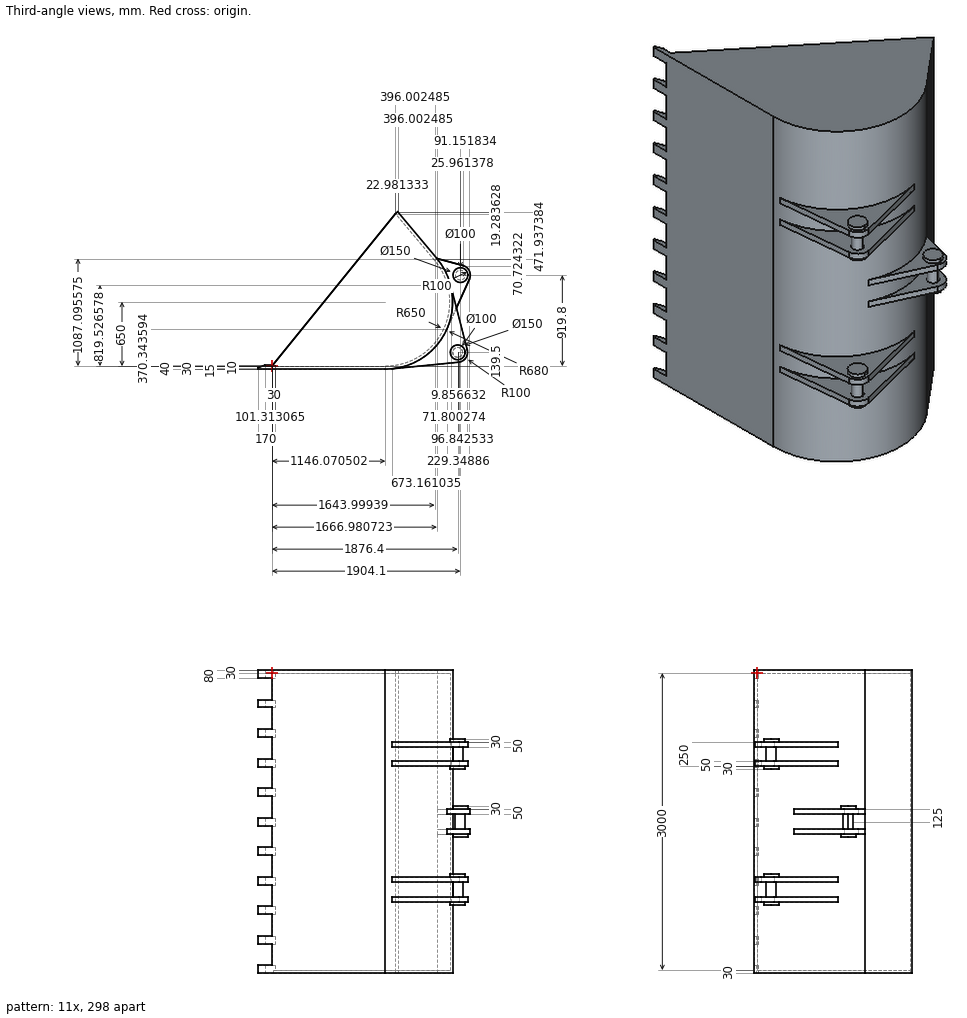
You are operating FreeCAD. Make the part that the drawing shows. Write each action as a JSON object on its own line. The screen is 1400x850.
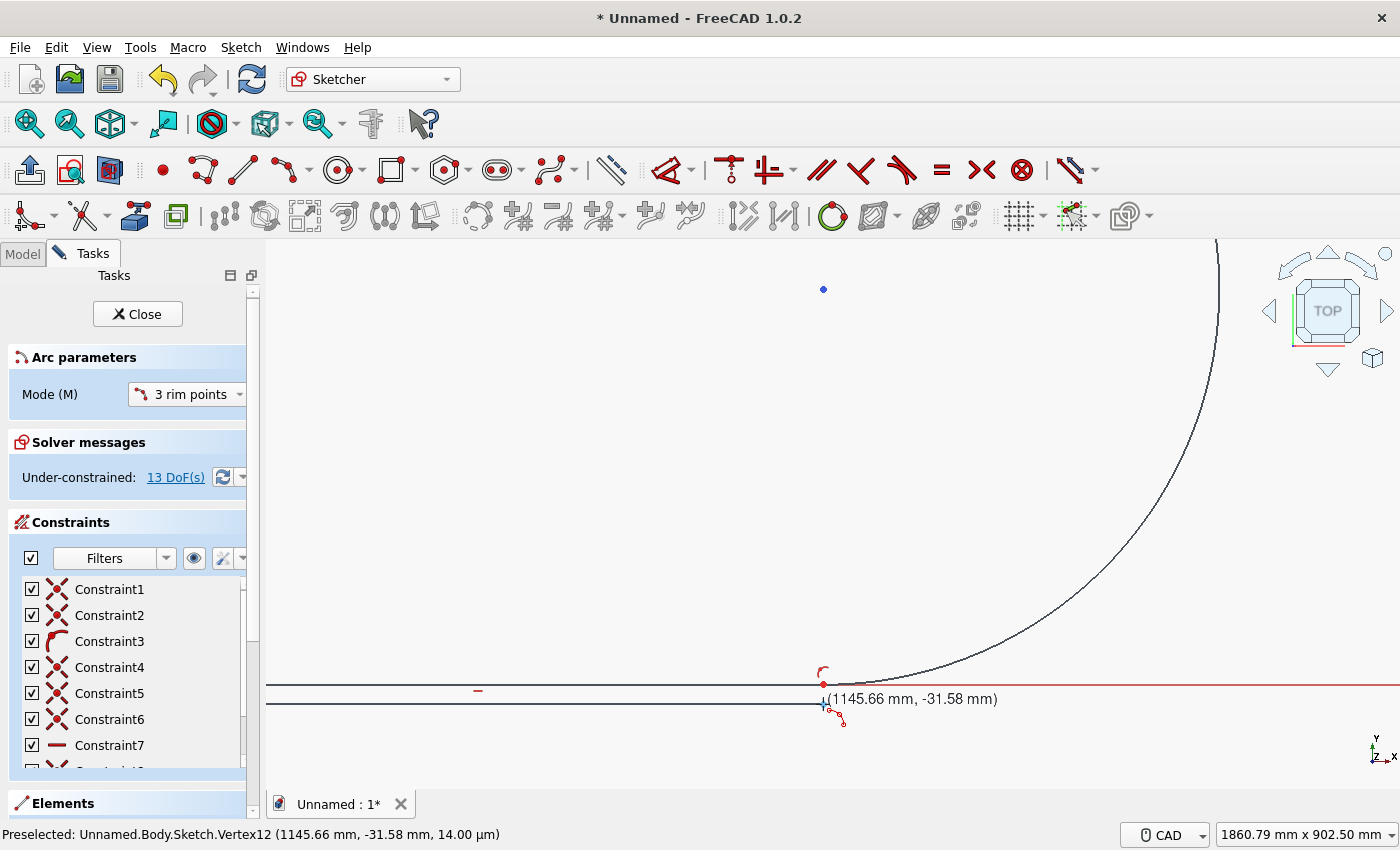
{"action": "scroll", "coordinate": [824, 686], "scroll_direction": "down", "scroll_amount": 5}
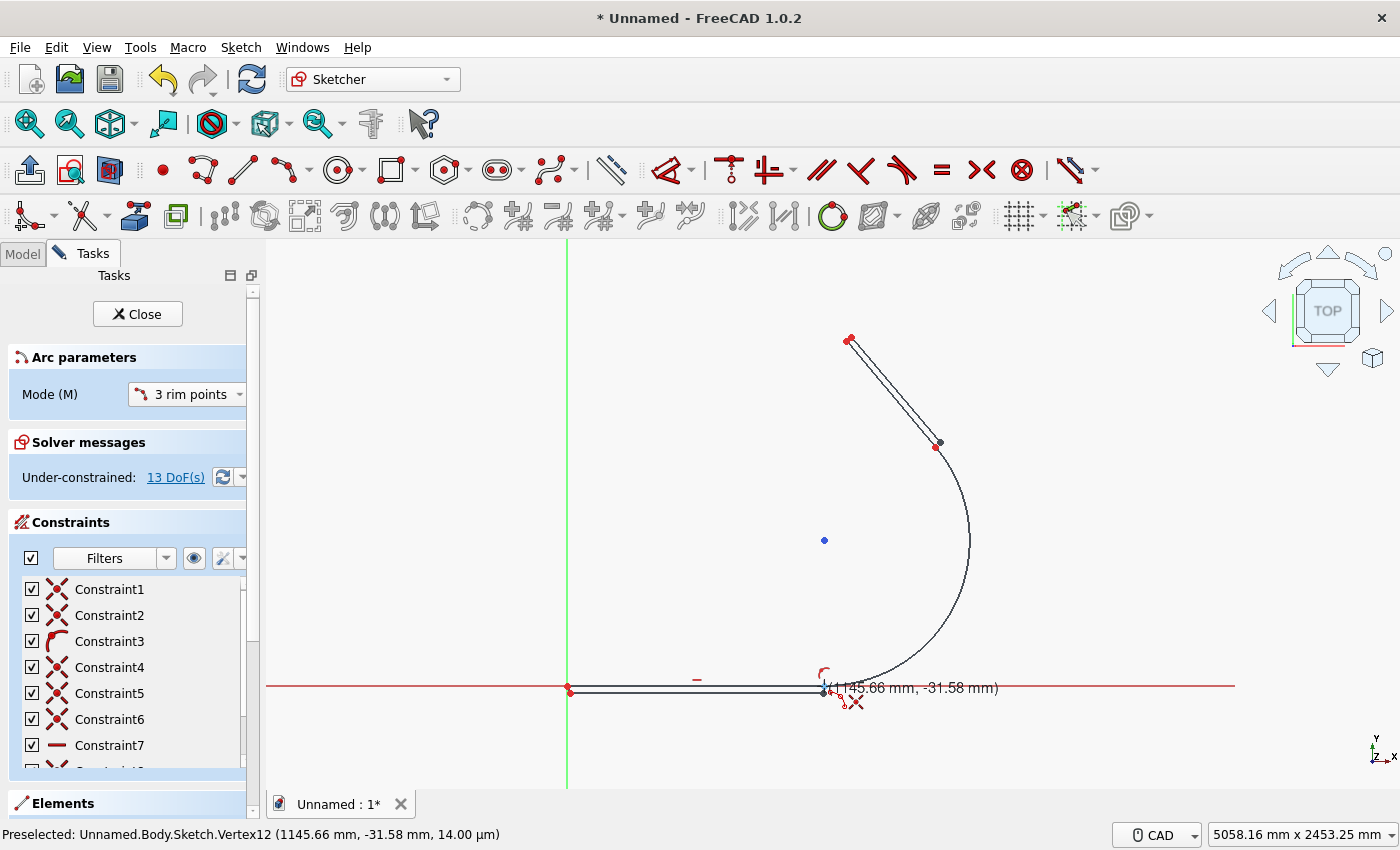
{"action": "scroll", "coordinate": [941, 442], "scroll_direction": "up", "scroll_amount": 5}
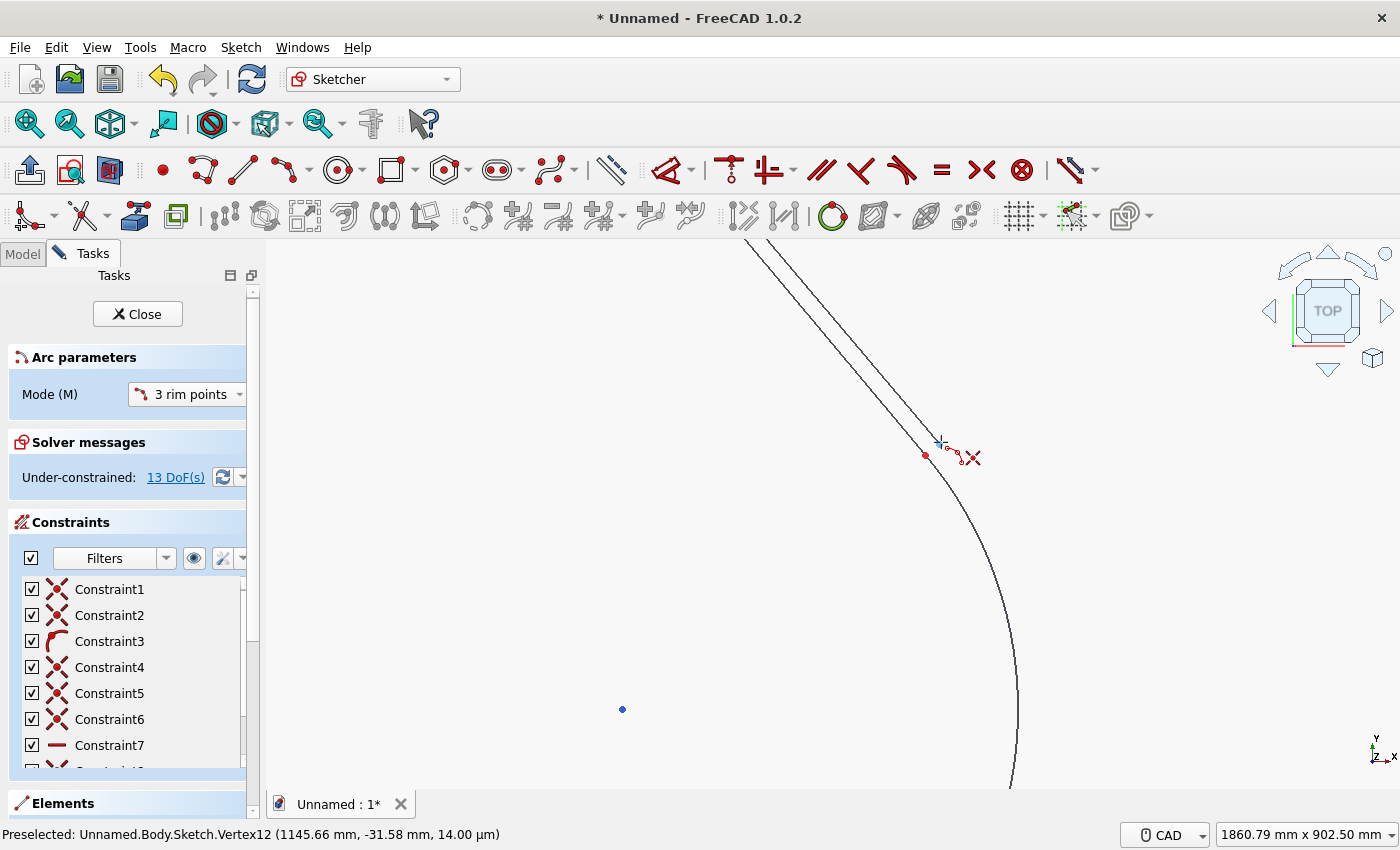
{"action": "left_click", "coordinate": [940, 444]}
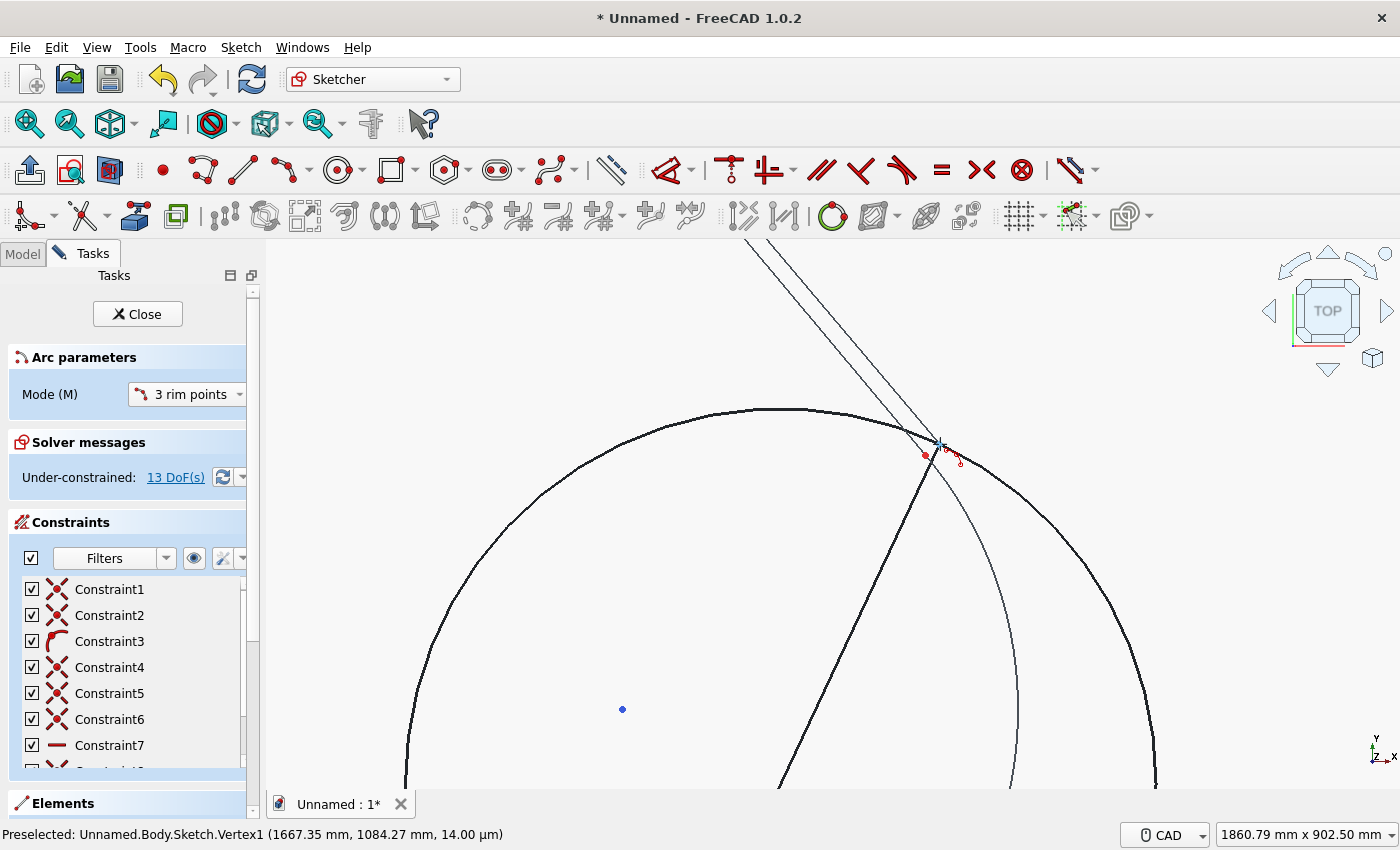
{"action": "scroll", "coordinate": [941, 441], "scroll_direction": "down", "scroll_amount": 5}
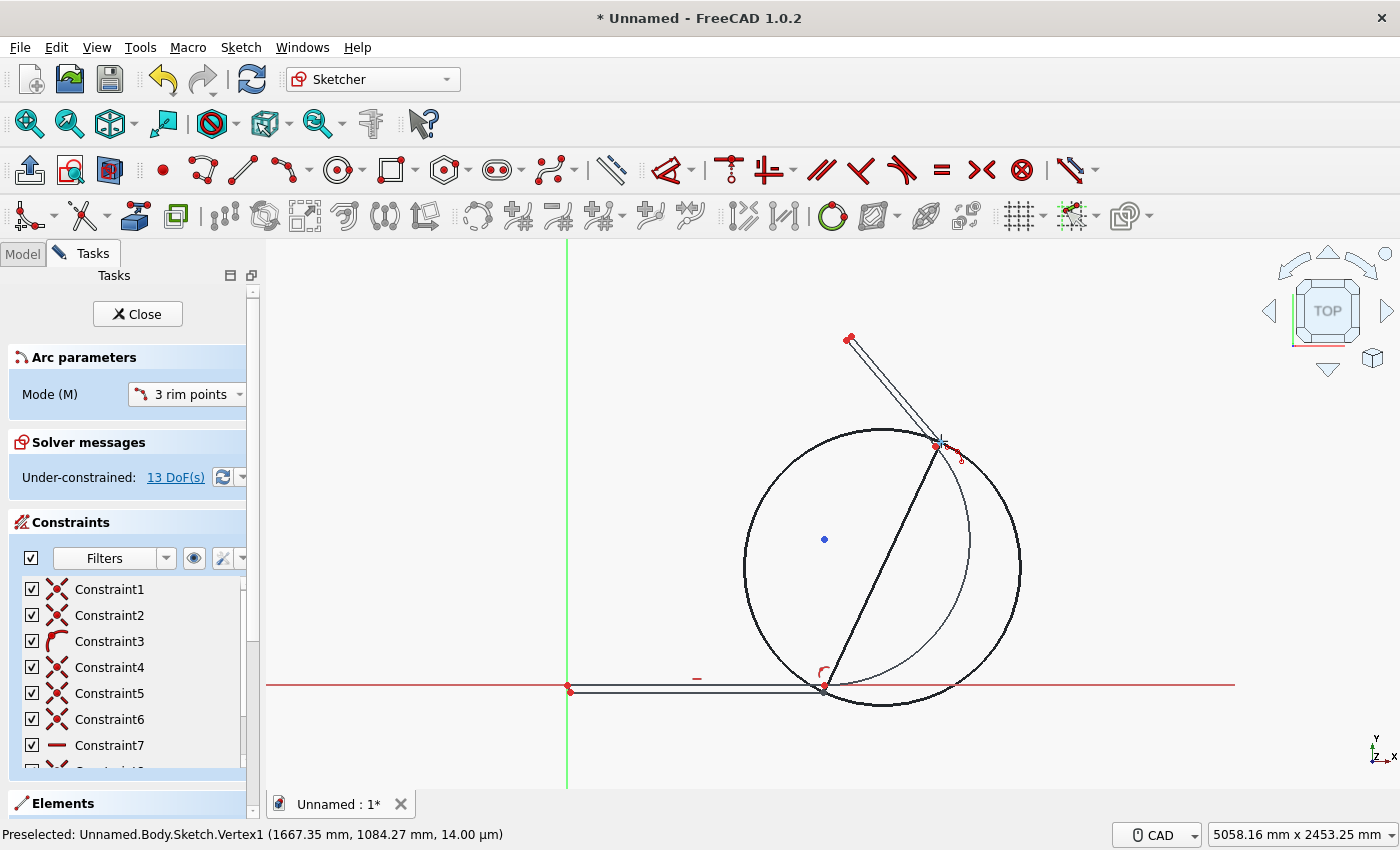
{"action": "scroll", "coordinate": [962, 604], "scroll_direction": "up", "scroll_amount": 5}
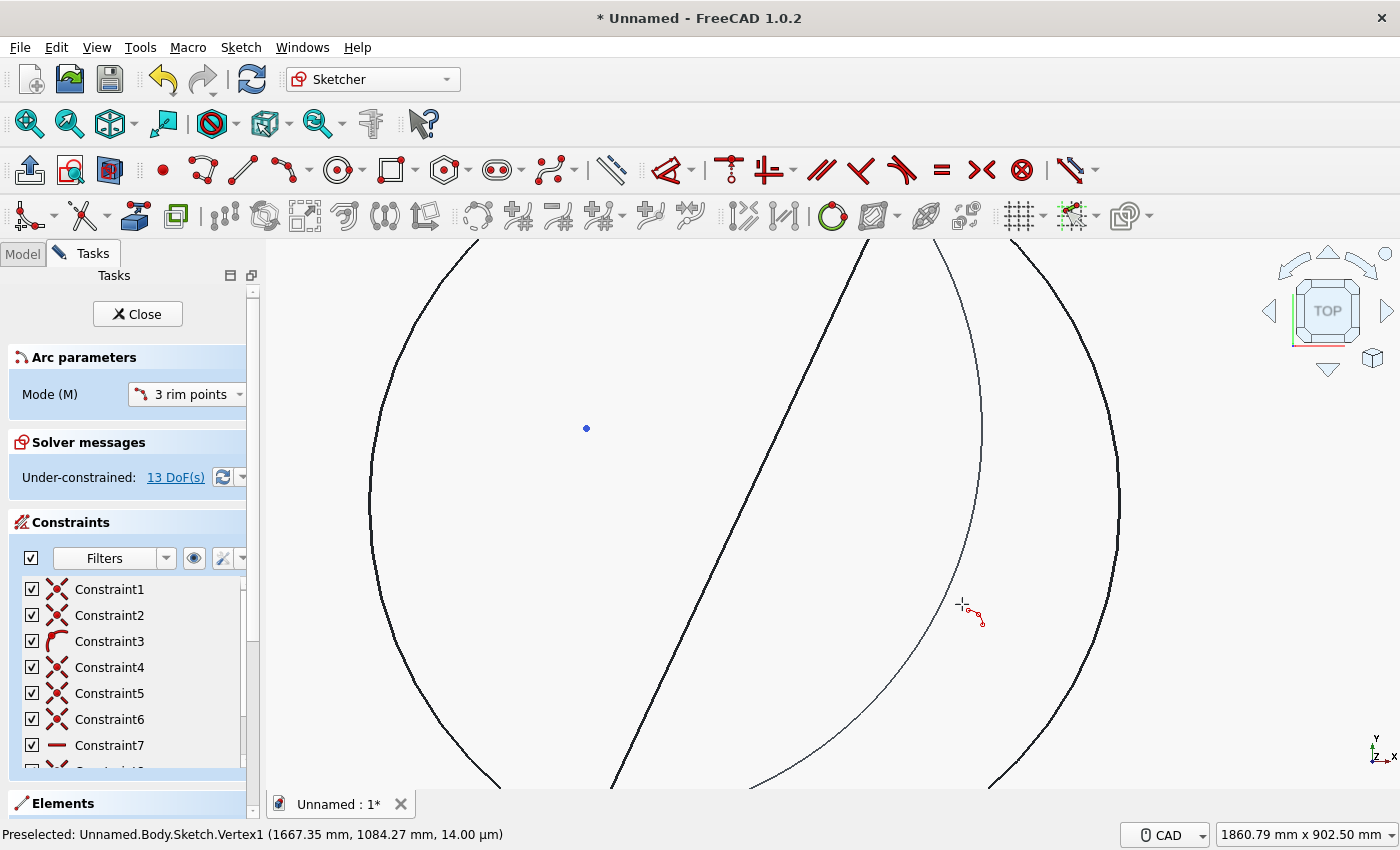
{"action": "left_click", "coordinate": [961, 603]}
{"action": "key", "text": "Escape"}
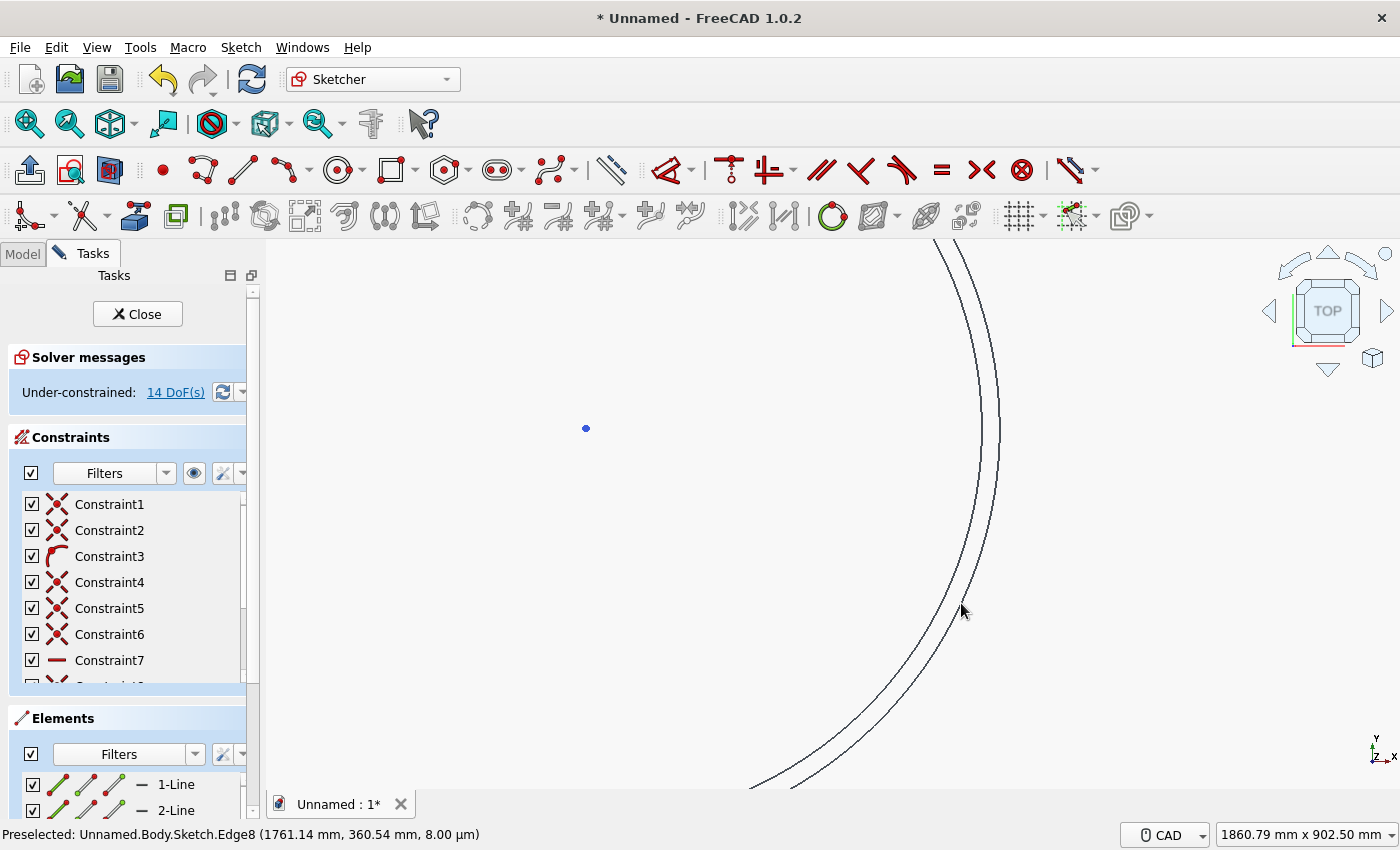
{"action": "scroll", "coordinate": [962, 605], "scroll_direction": "down", "scroll_amount": 5}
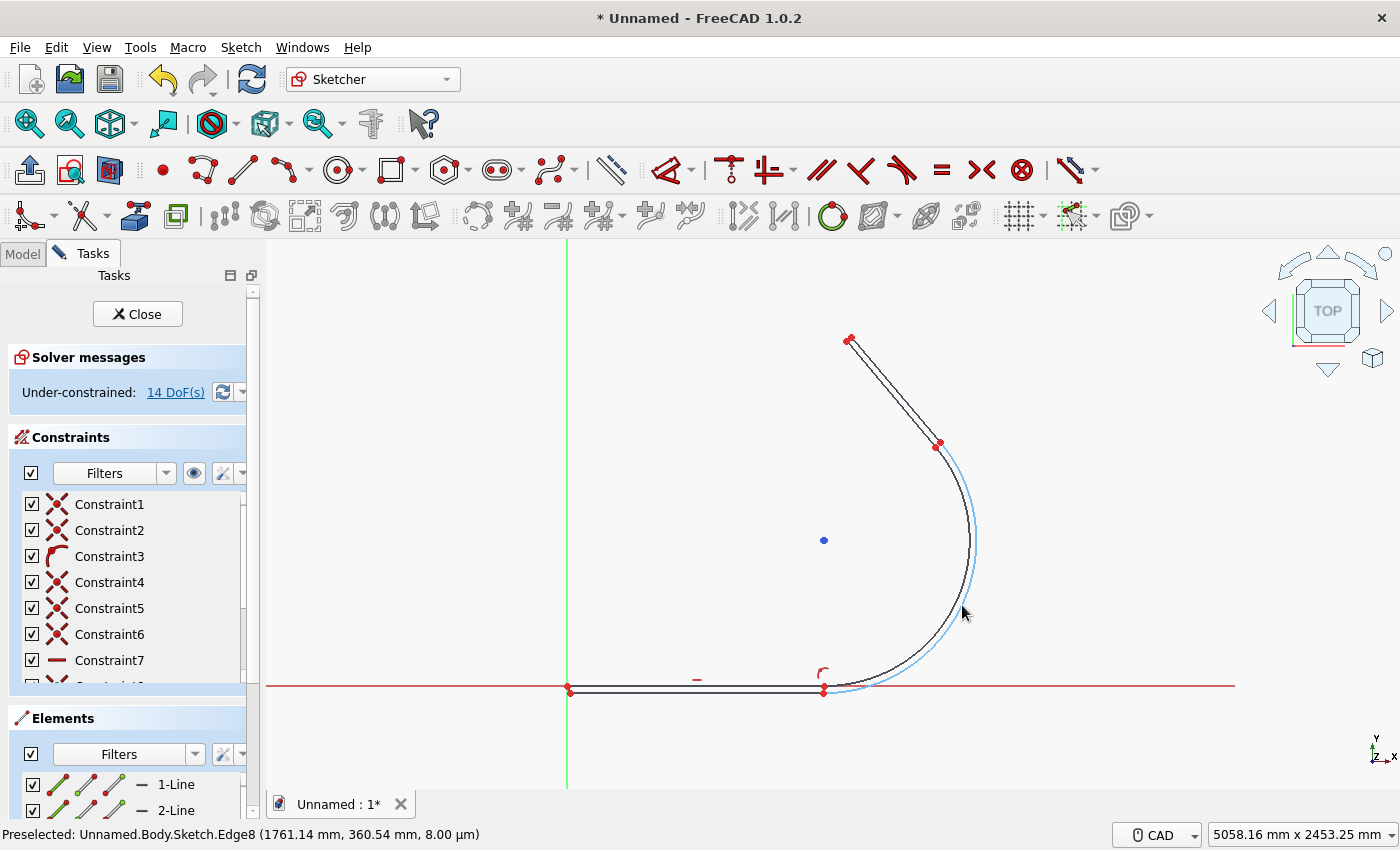
{"action": "scroll", "coordinate": [568, 689], "scroll_direction": "up", "scroll_amount": 8}